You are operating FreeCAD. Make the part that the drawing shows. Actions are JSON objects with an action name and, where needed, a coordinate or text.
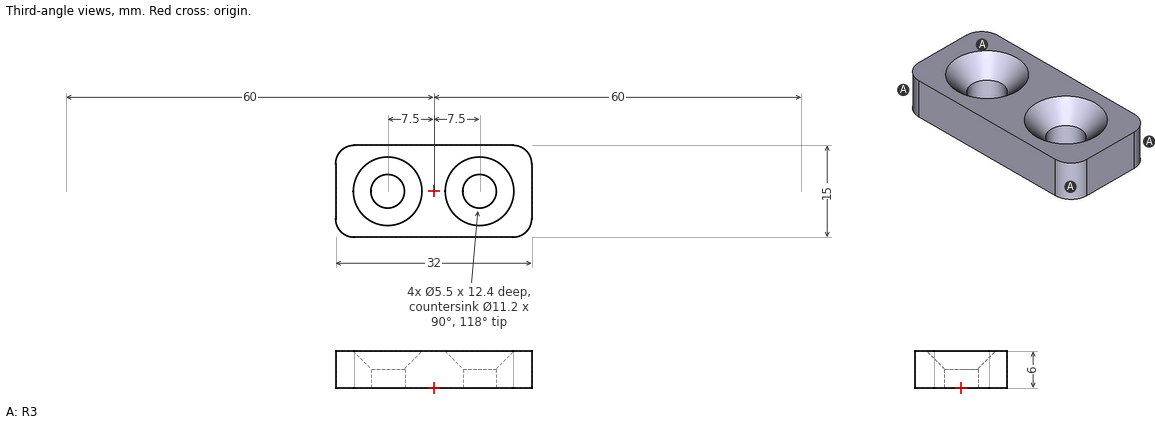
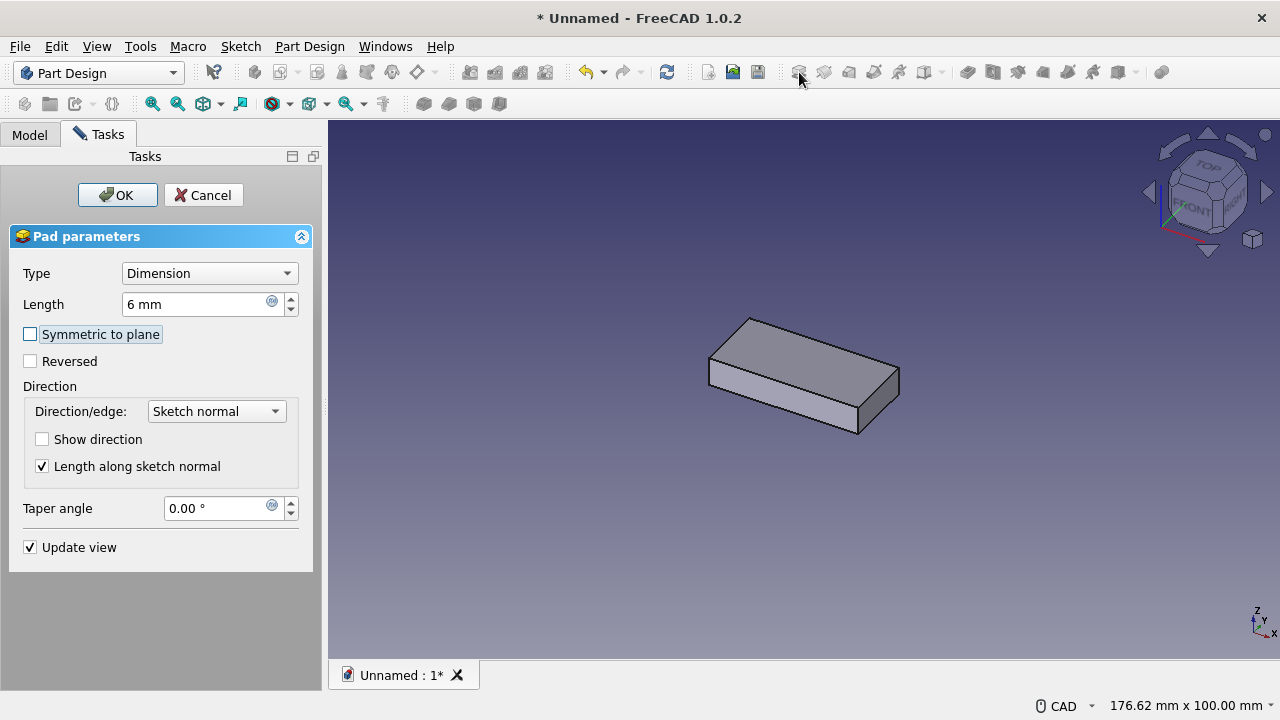
{"action": "left_click", "coordinate": [118, 195]}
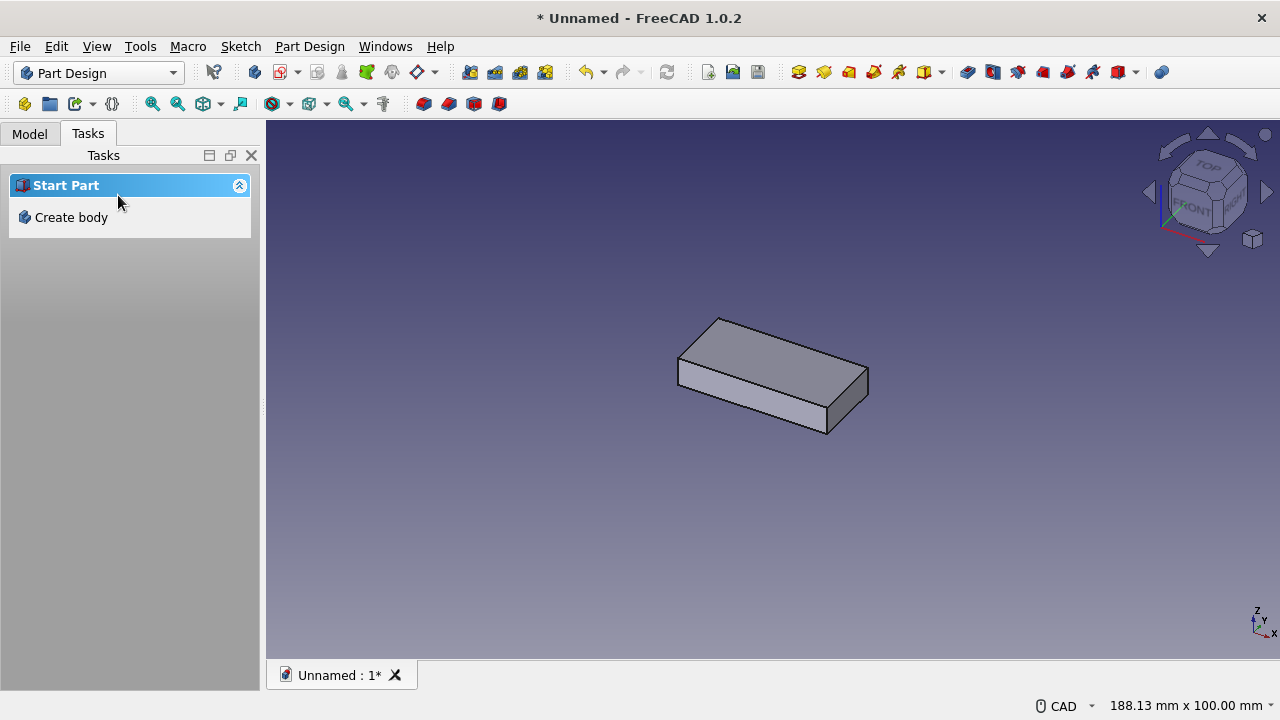
{"action": "left_click", "coordinate": [153, 104]}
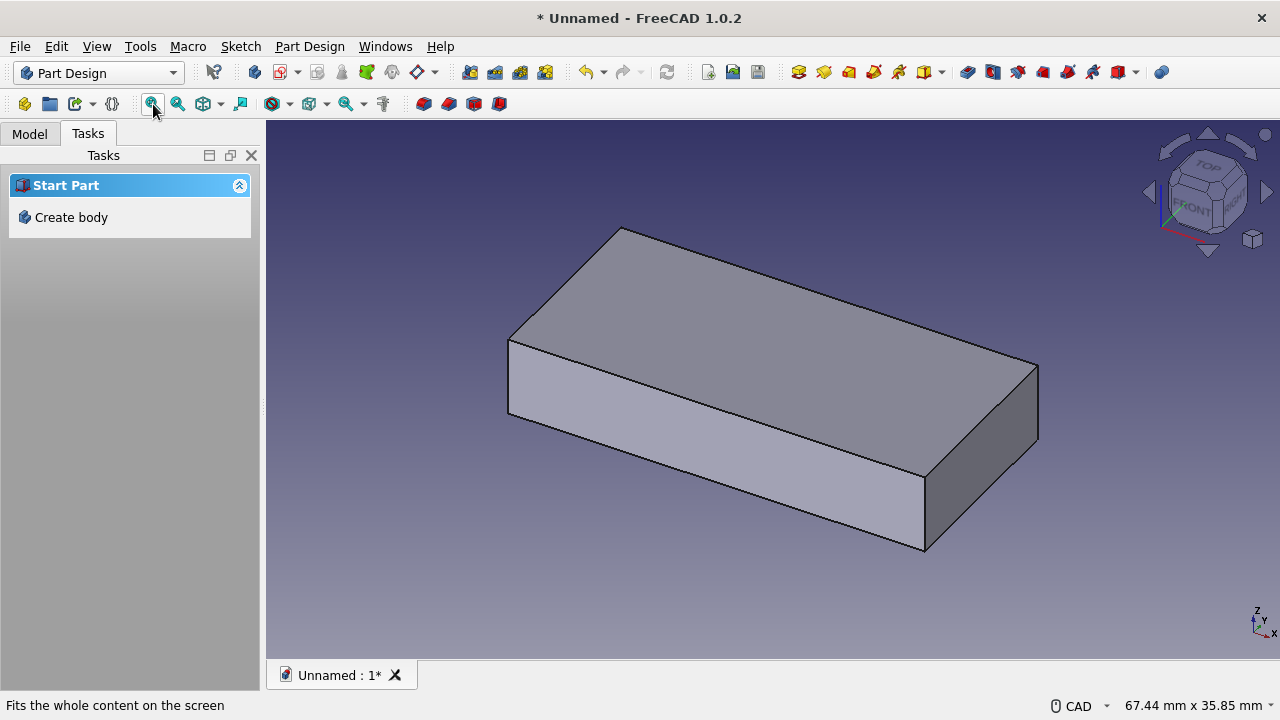
{"action": "left_click", "coordinate": [833, 371]}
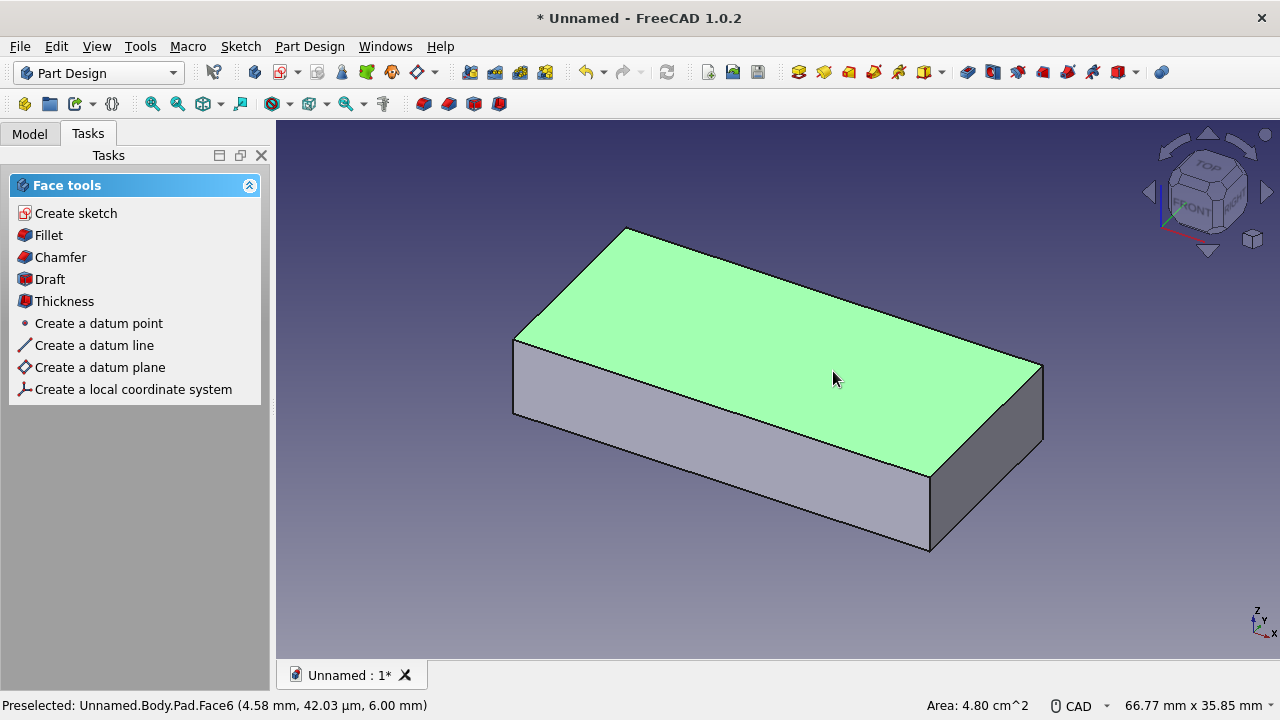
{"action": "left_click", "coordinate": [280, 72]}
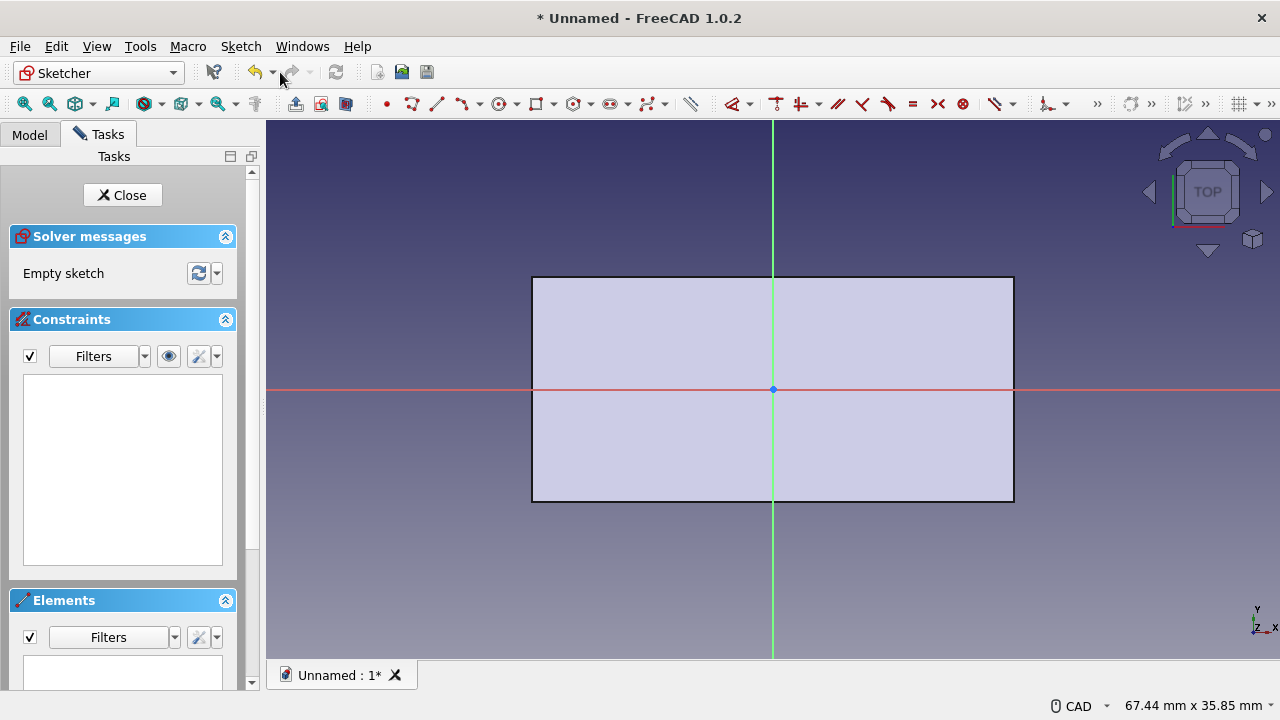
{"action": "scroll", "coordinate": [675, 389], "scroll_direction": "down", "scroll_amount": 6}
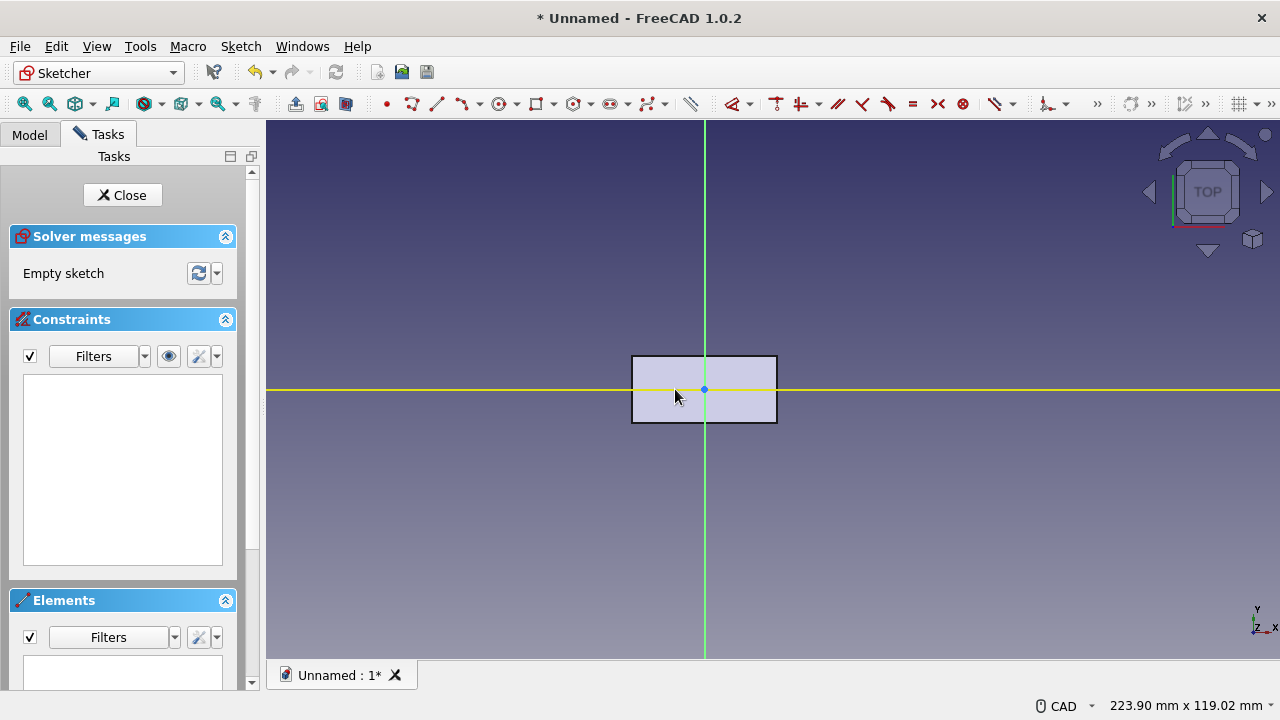
{"action": "left_click", "coordinate": [498, 104]}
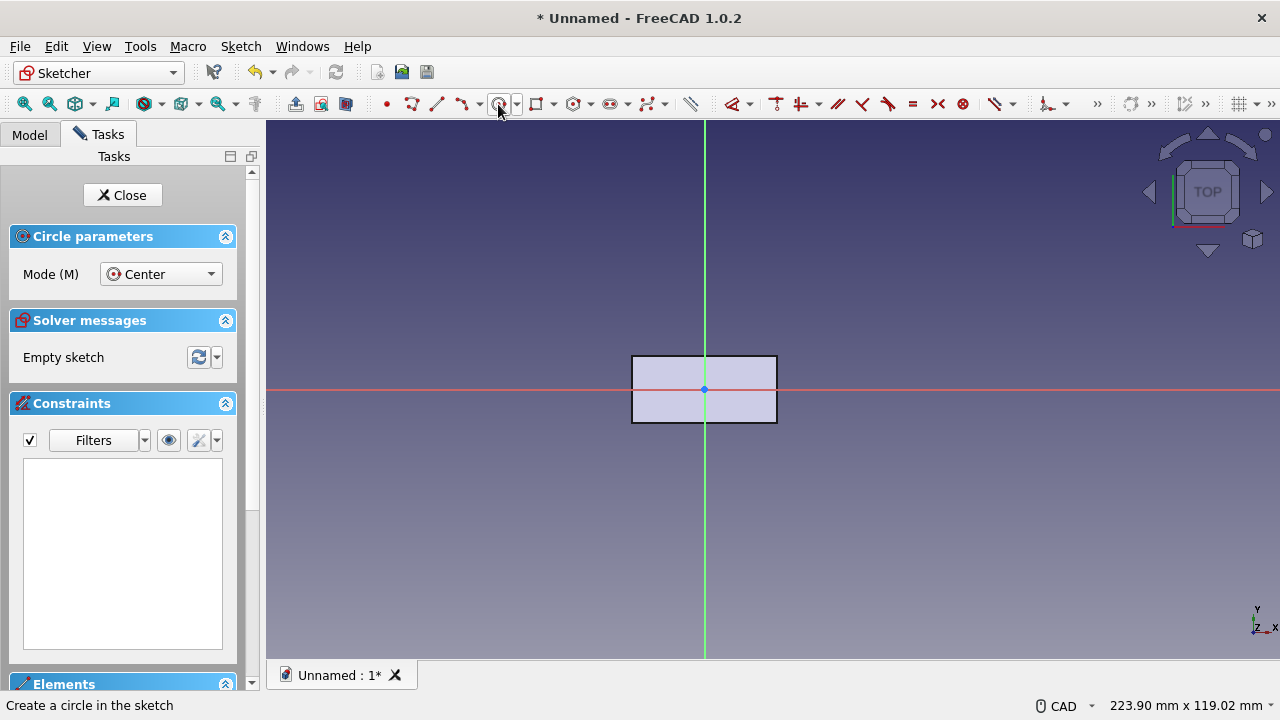
{"action": "scroll", "coordinate": [739, 390], "scroll_direction": "up", "scroll_amount": 3}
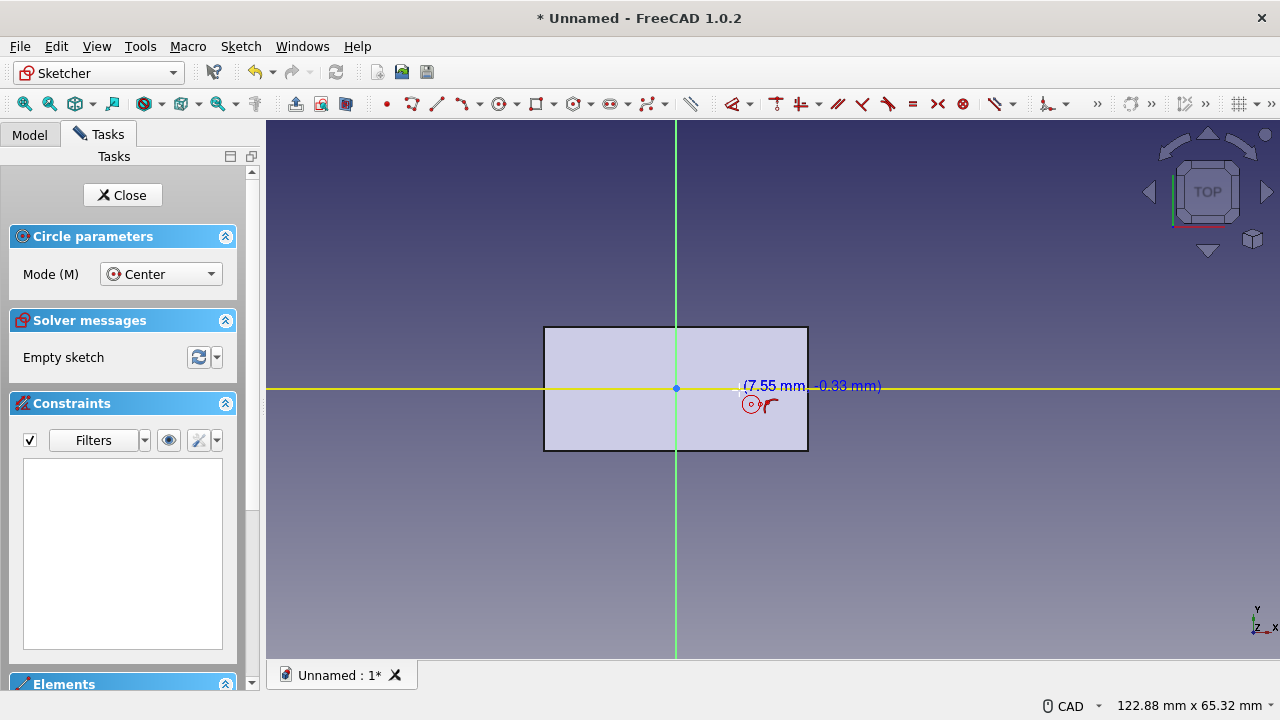
{"action": "left_click", "coordinate": [738, 389]}
{"action": "mouse_move", "coordinate": [754, 373]}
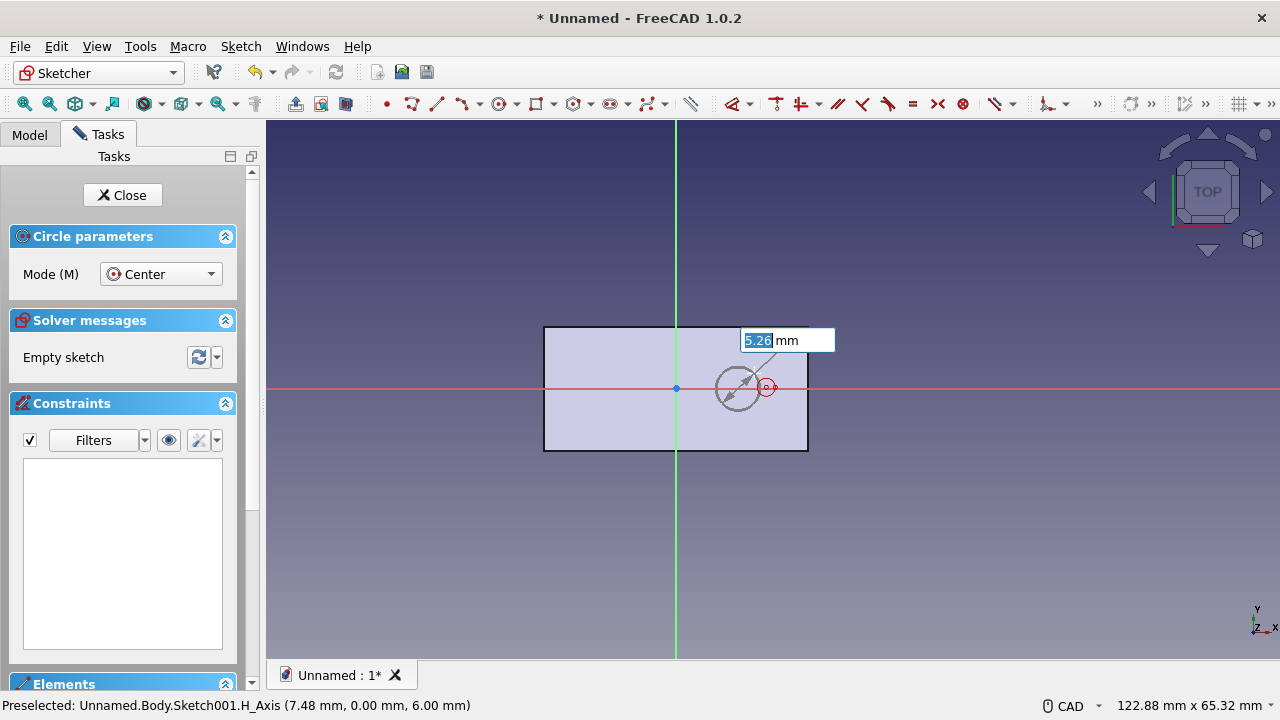
{"action": "type", "text": "5.5"}
{"action": "key", "text": "Return"}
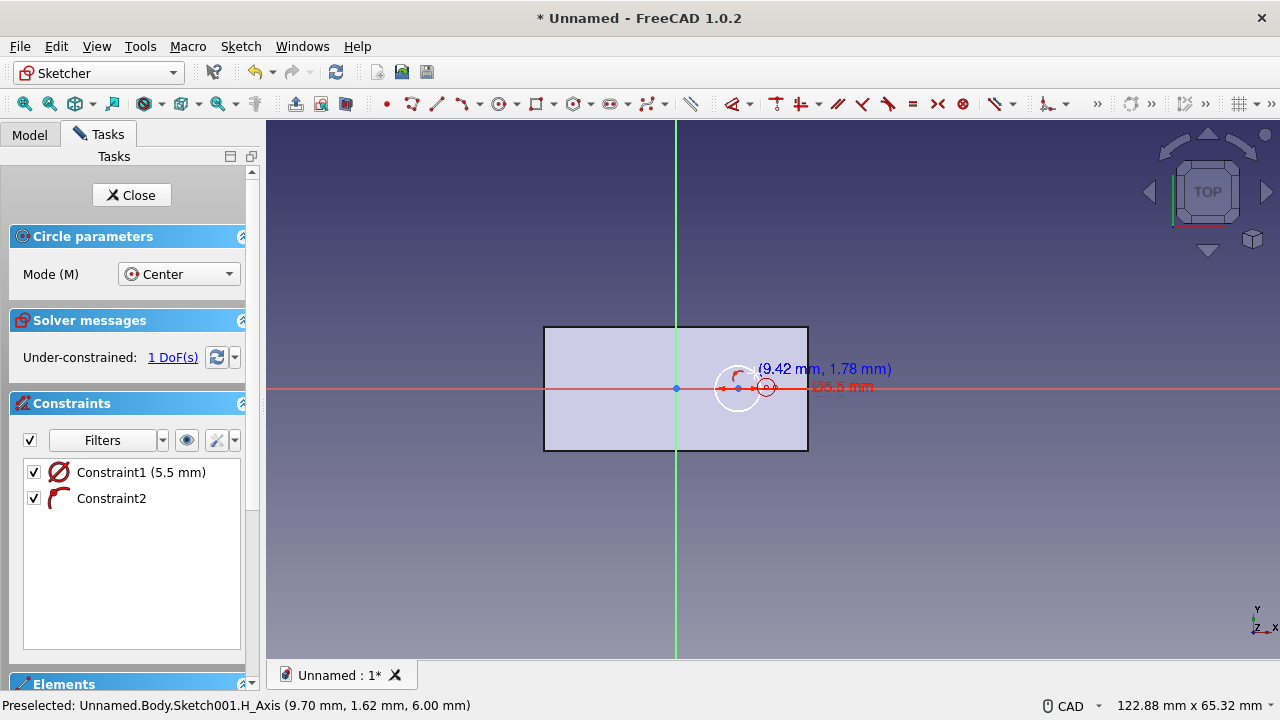
{"action": "scroll", "coordinate": [739, 391], "scroll_direction": "down", "scroll_amount": 3}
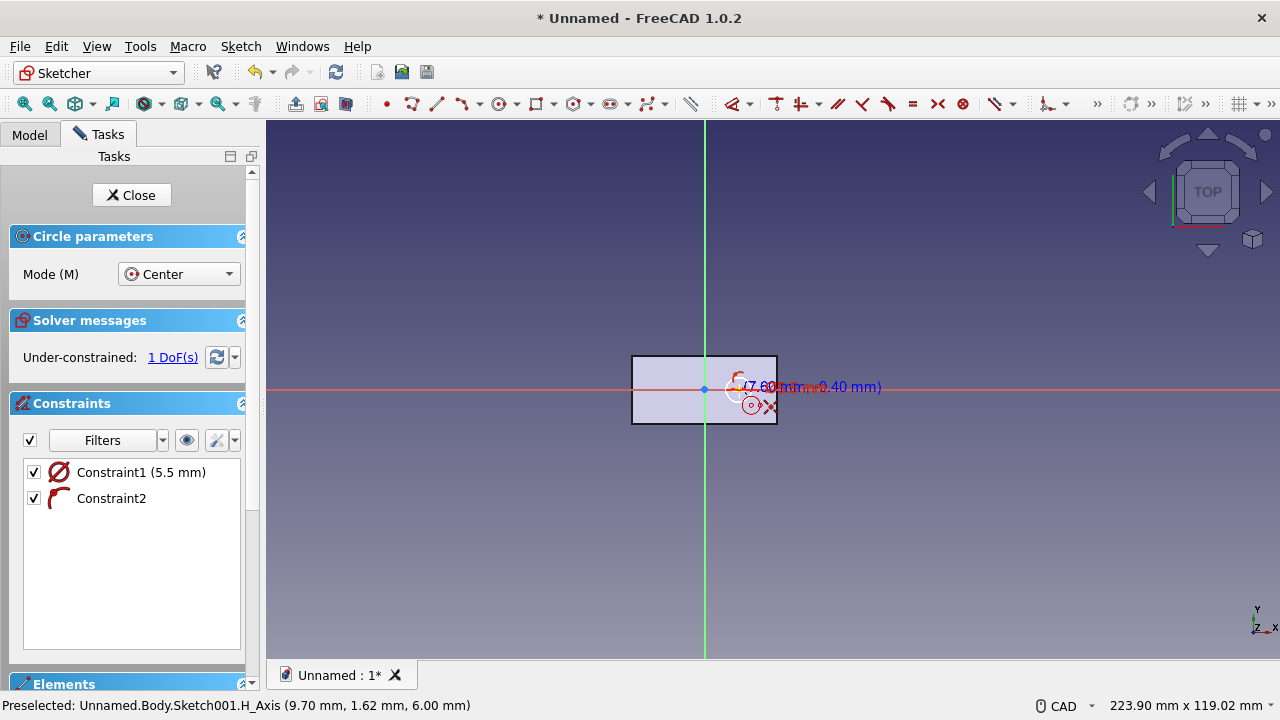
{"action": "scroll", "coordinate": [977, 390], "scroll_direction": "up", "scroll_amount": 3}